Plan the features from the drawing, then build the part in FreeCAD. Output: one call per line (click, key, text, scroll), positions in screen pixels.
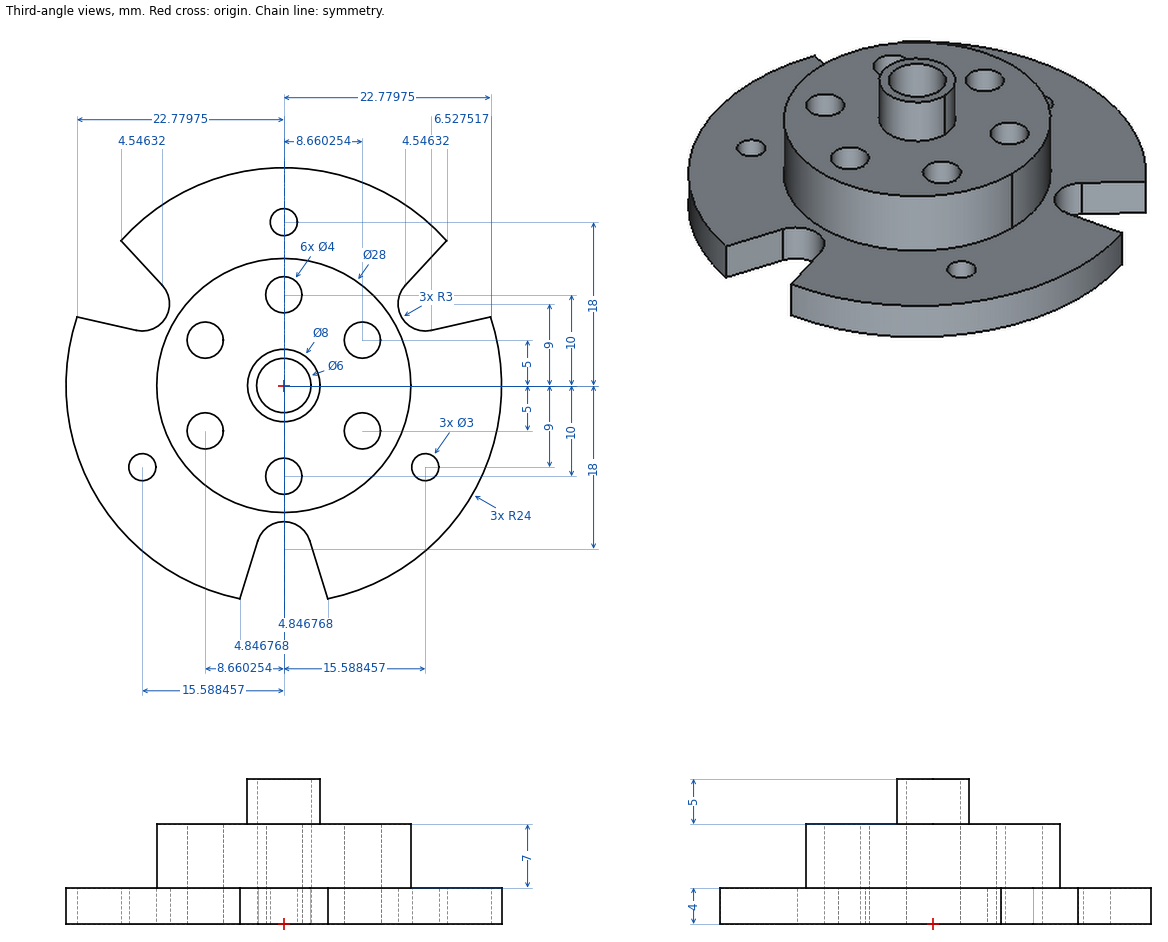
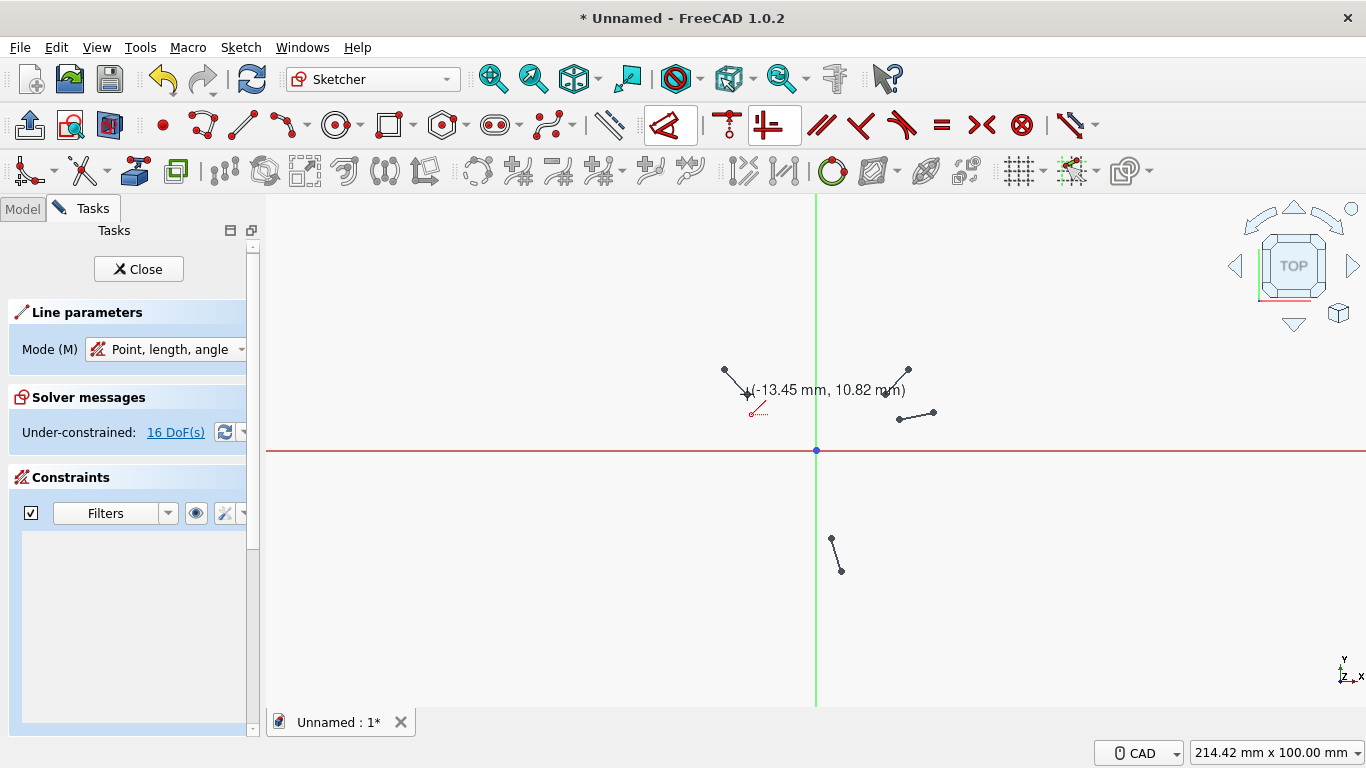
click(733, 419)
click(699, 412)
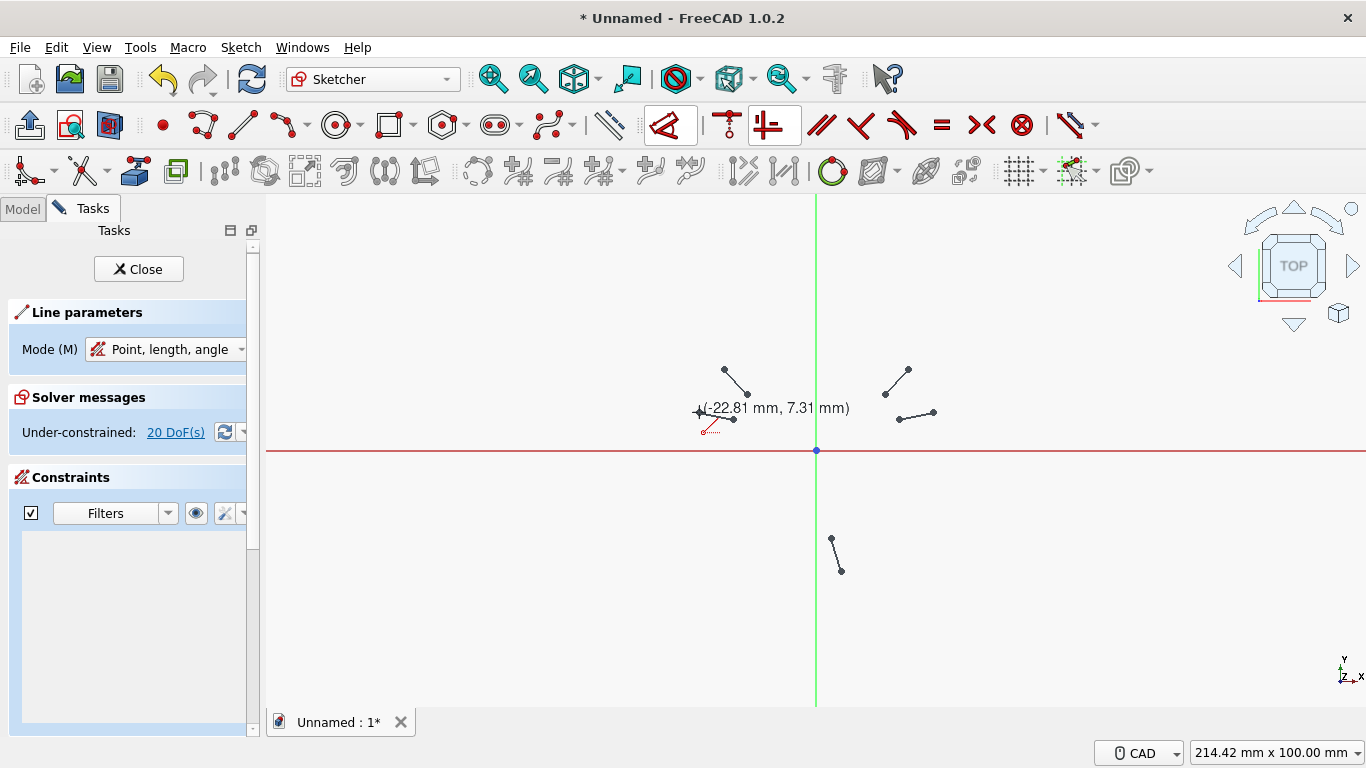
click(791, 571)
click(801, 538)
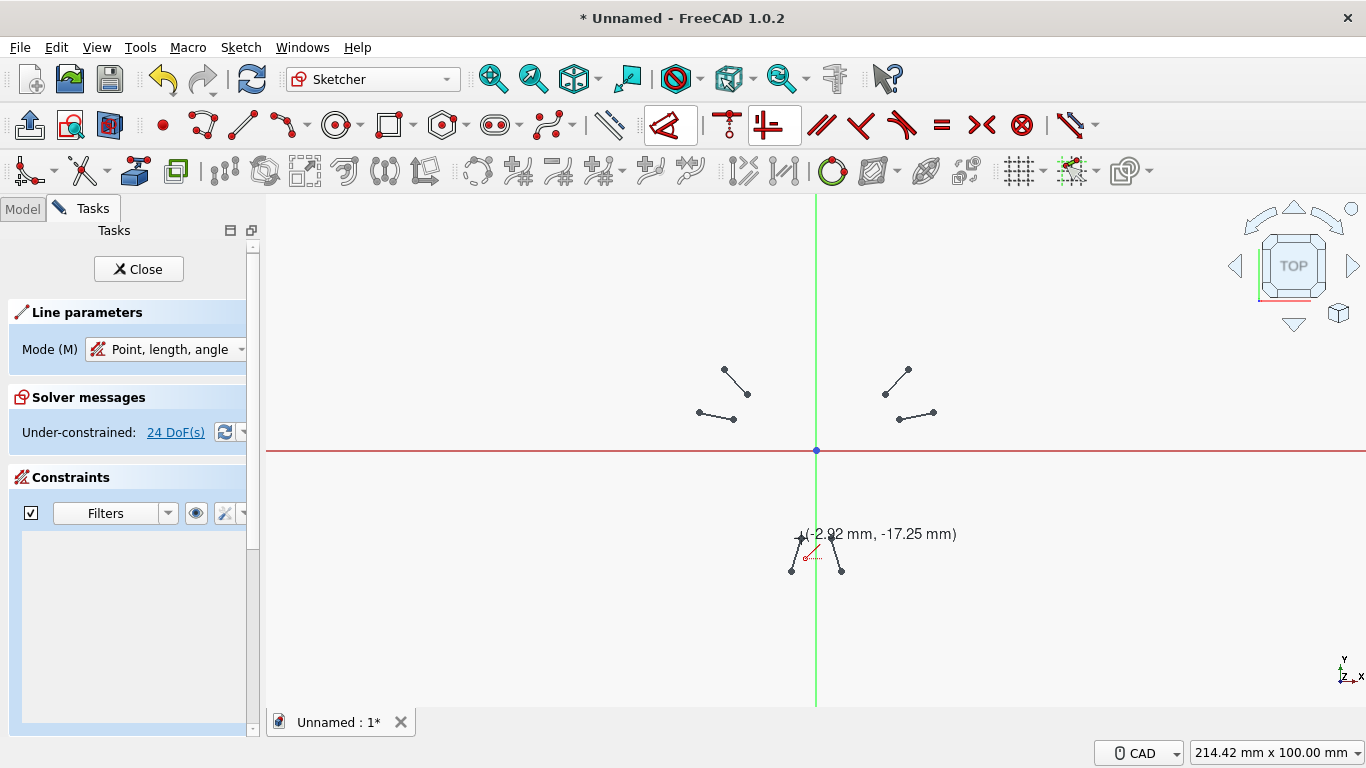
key(g)
key(3)
key(a)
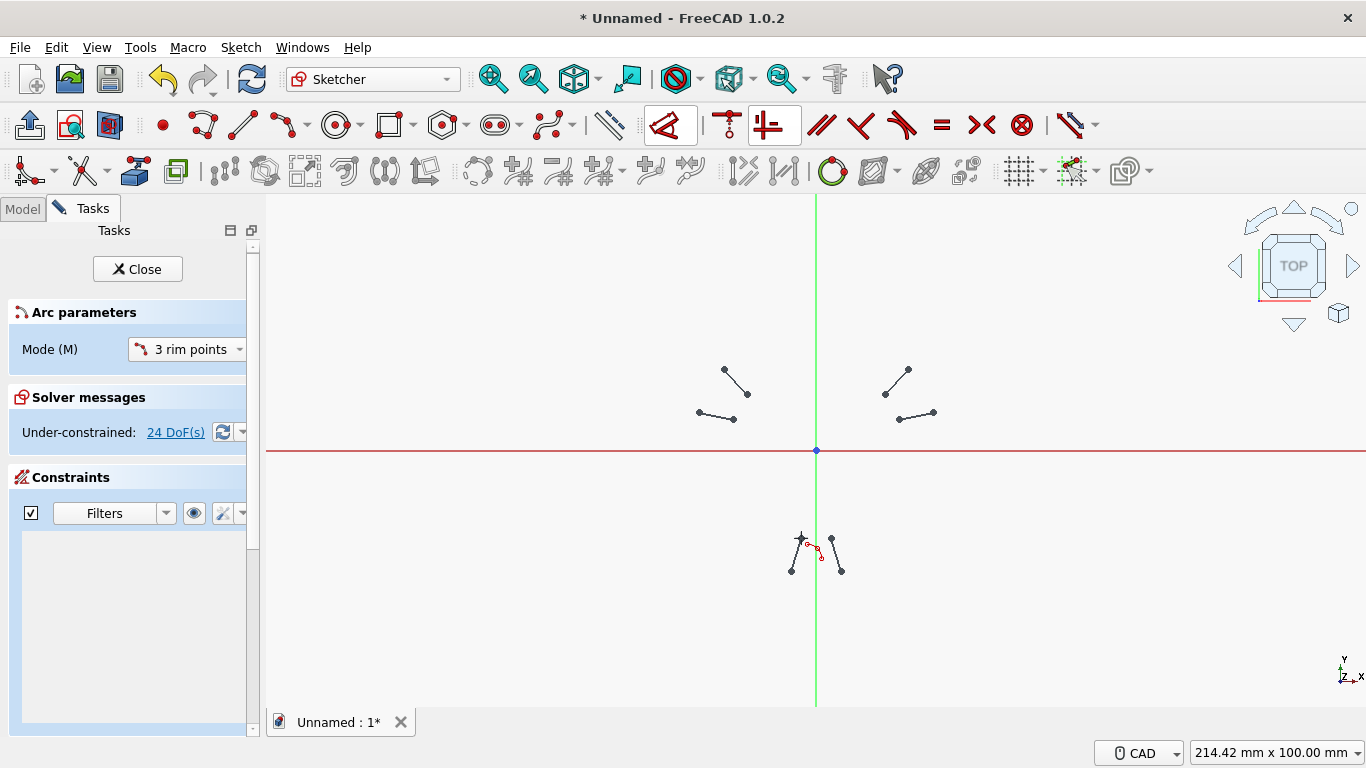
click(841, 572)
click(933, 413)
click(923, 512)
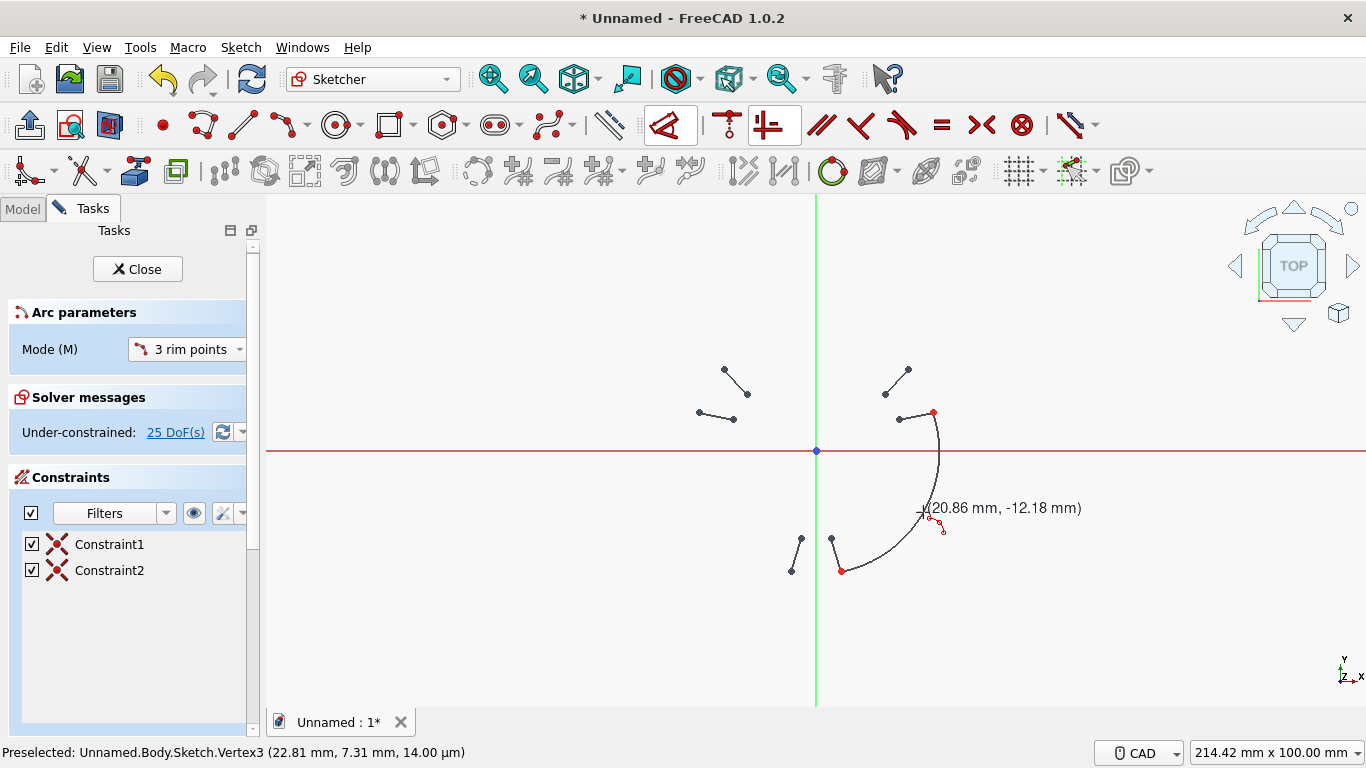
click(899, 420)
click(885, 395)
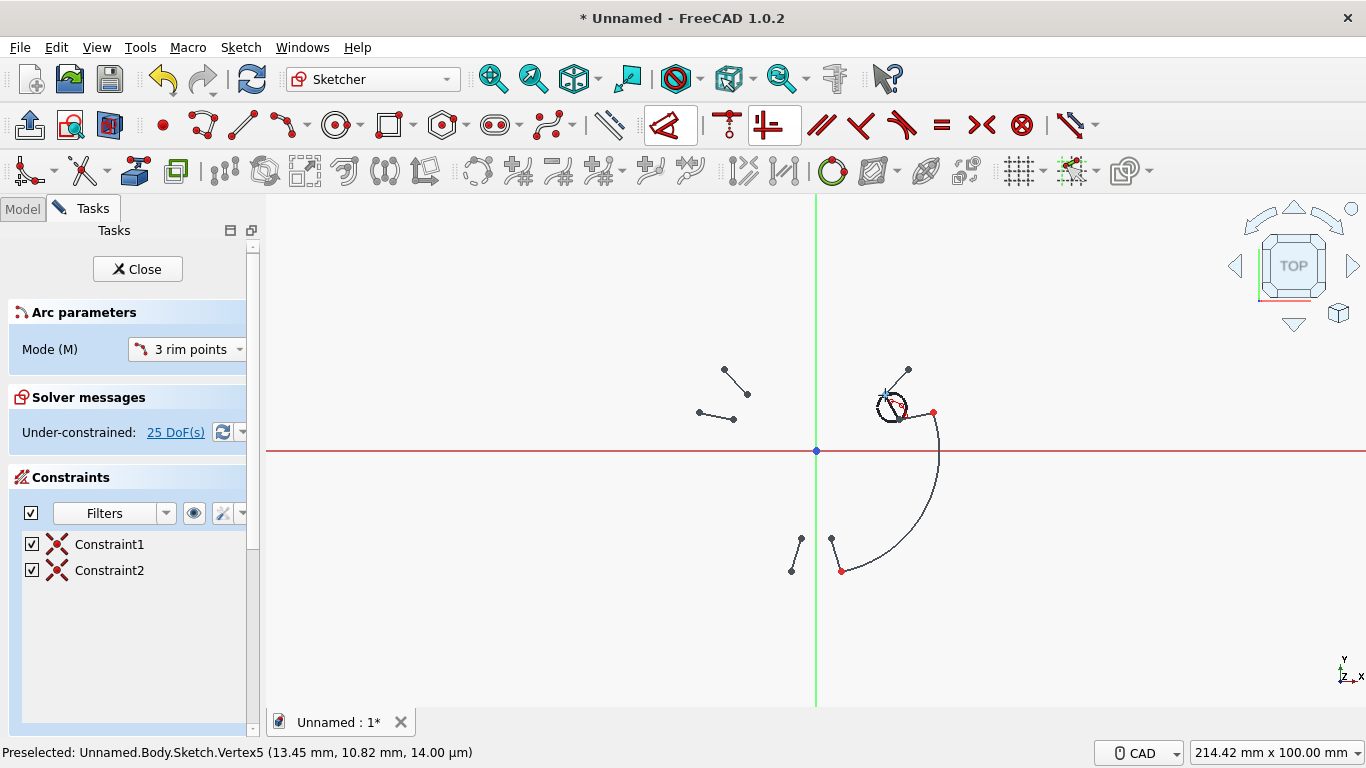
scroll(883, 412, up, 2)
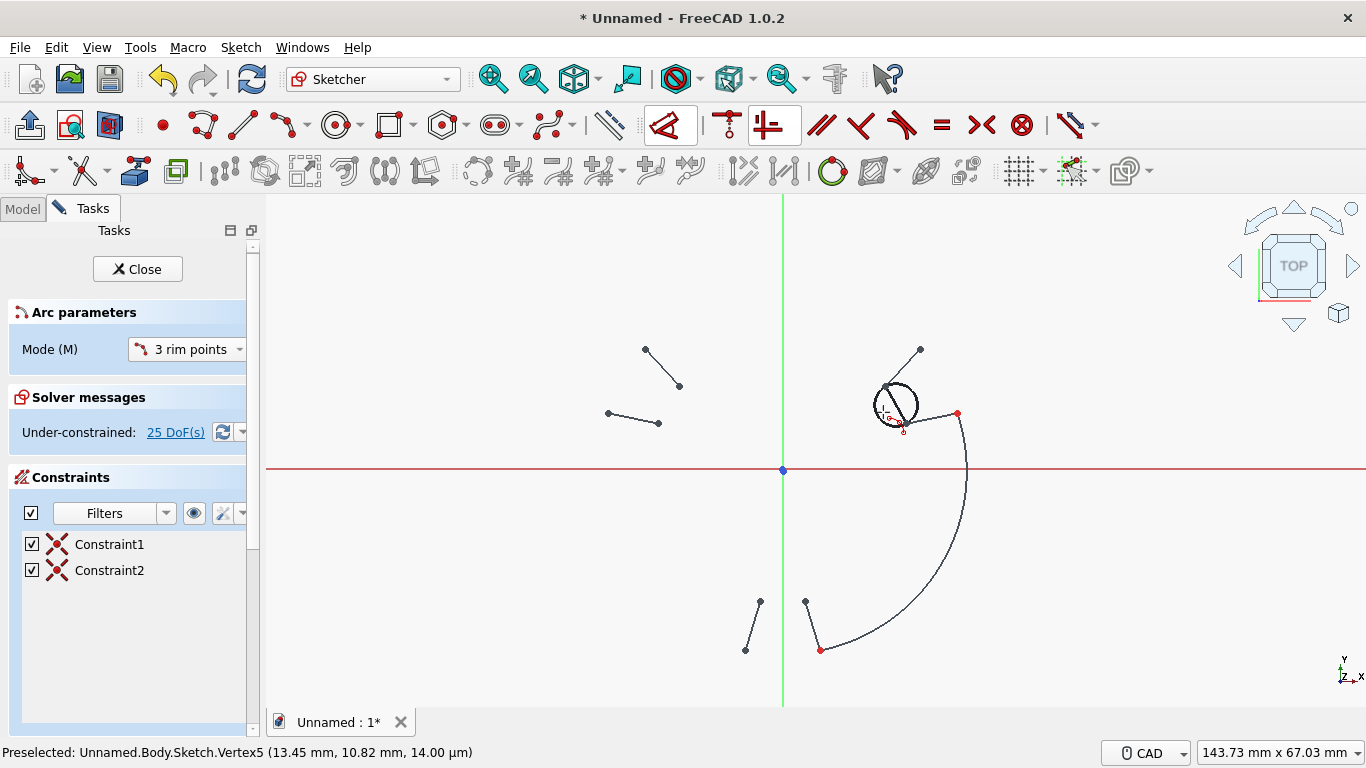
click(882, 412)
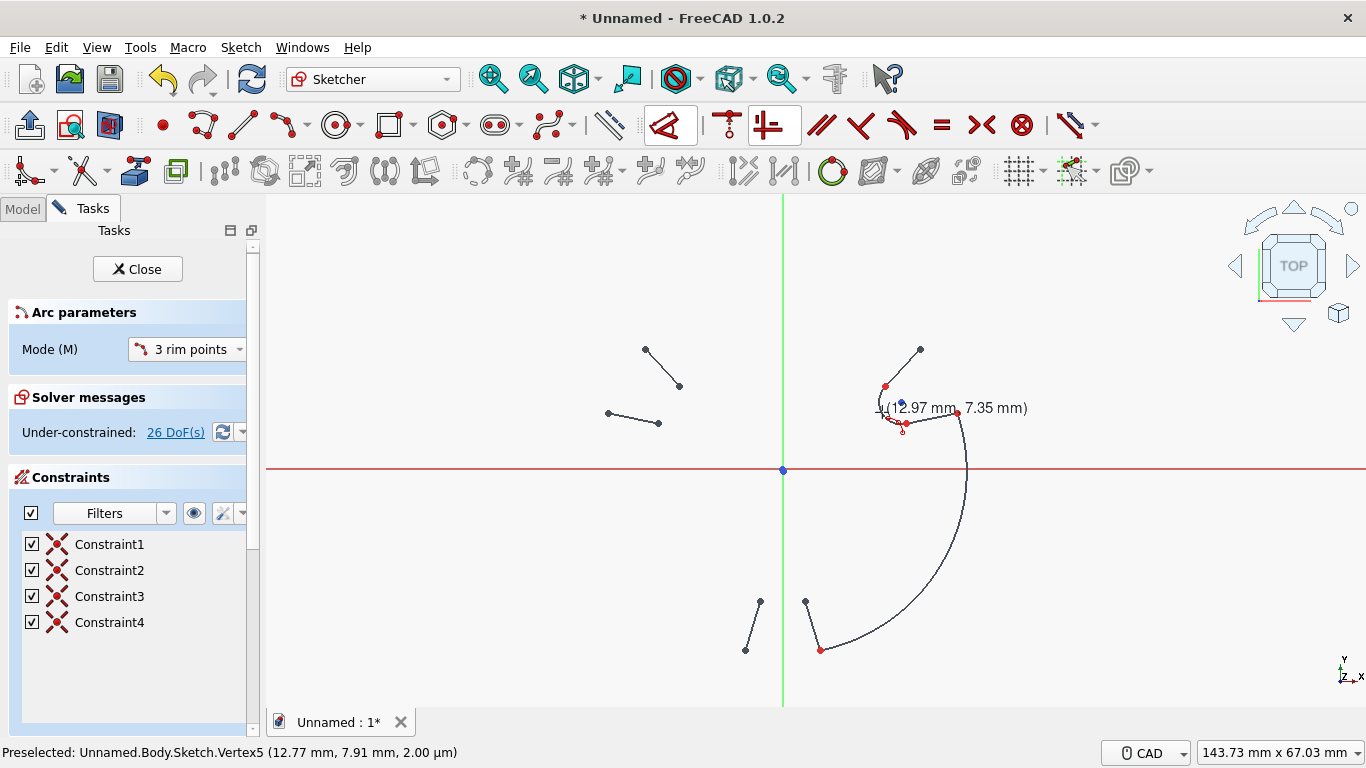
click(920, 349)
click(646, 349)
click(814, 288)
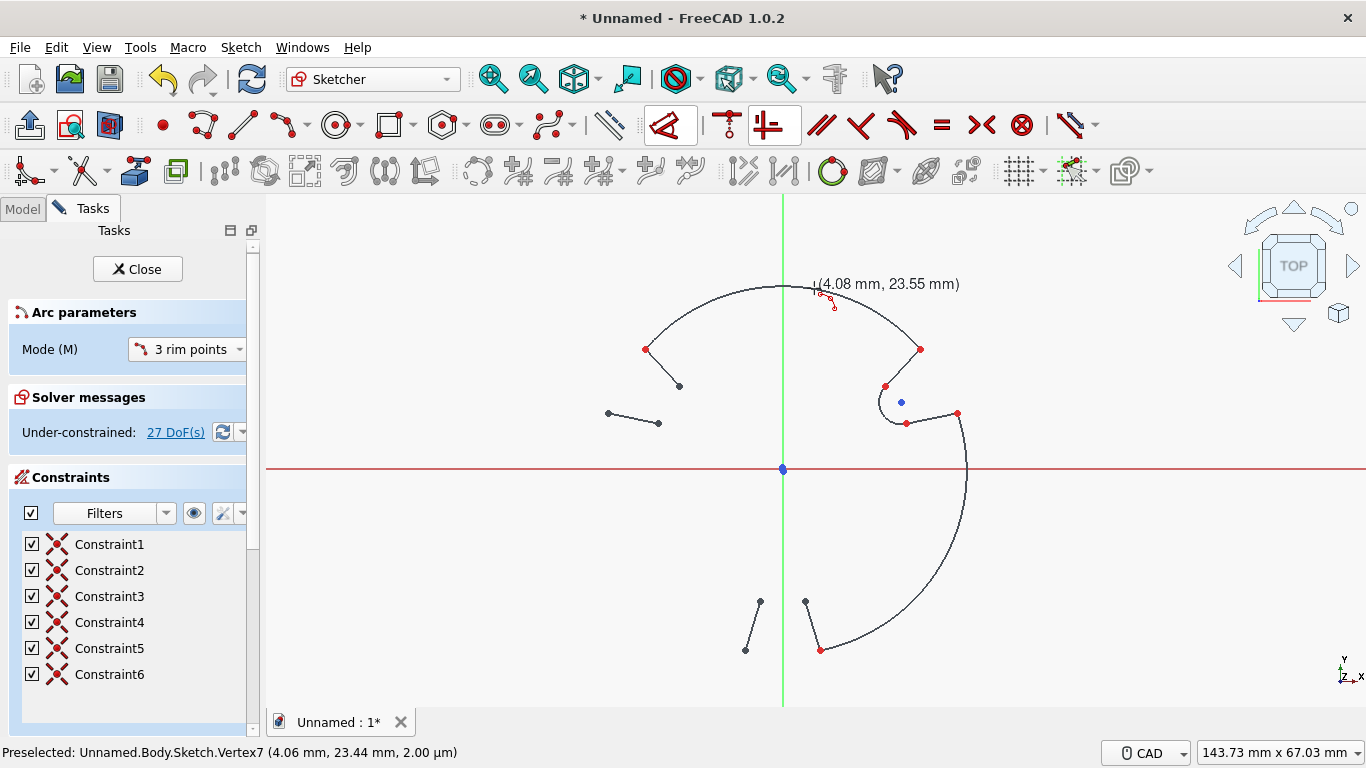
click(680, 386)
click(659, 424)
click(683, 412)